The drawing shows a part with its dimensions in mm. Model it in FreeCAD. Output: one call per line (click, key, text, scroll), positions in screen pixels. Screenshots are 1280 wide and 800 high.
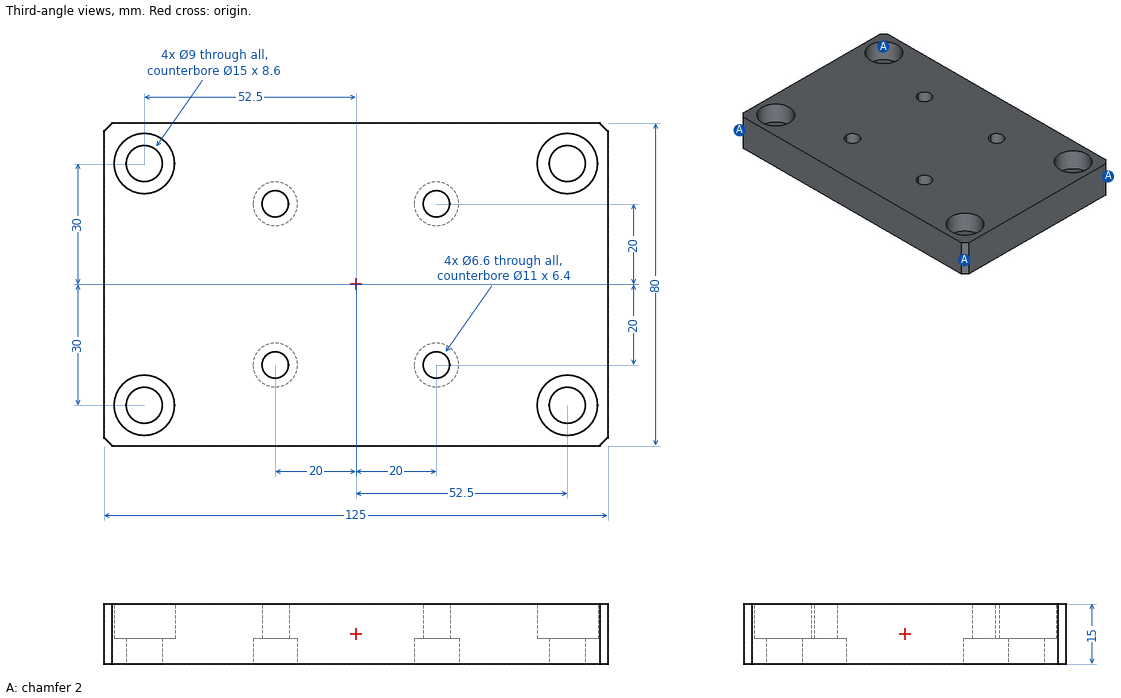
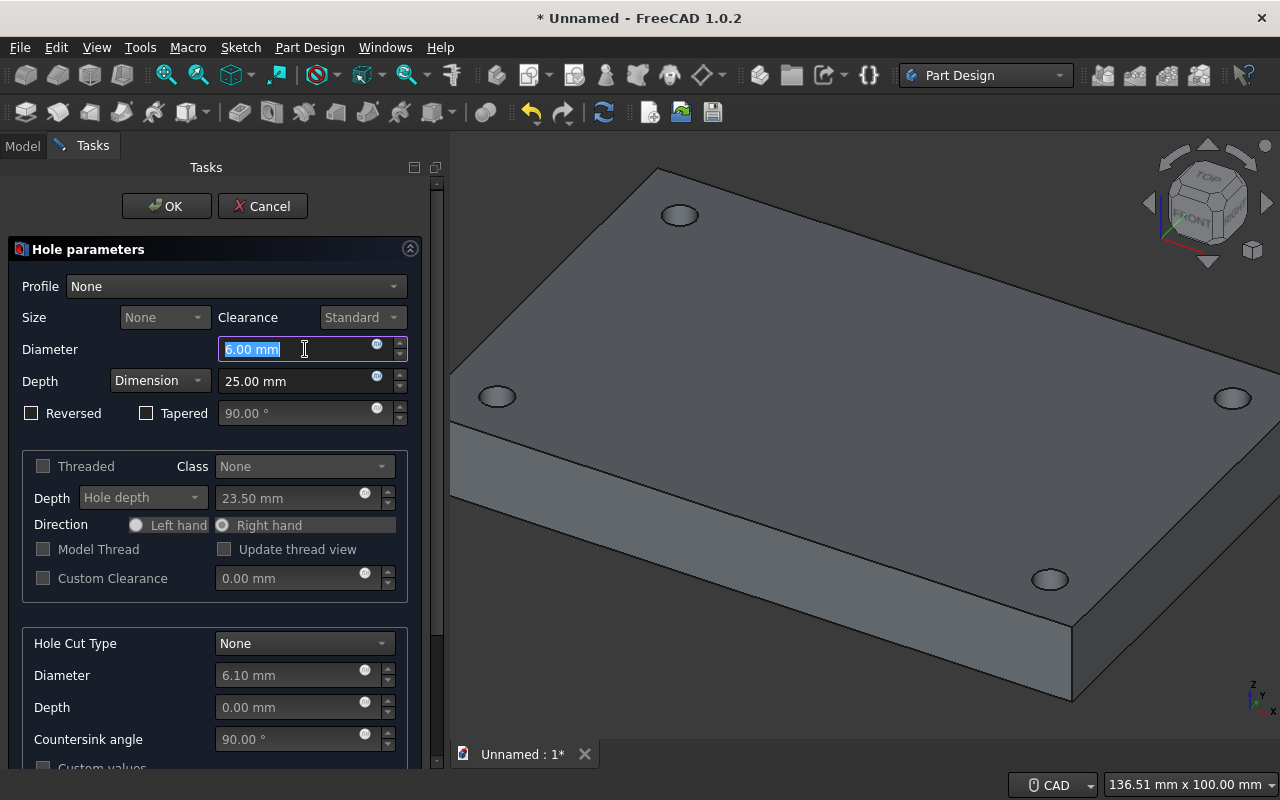
text(9)
key(Tab)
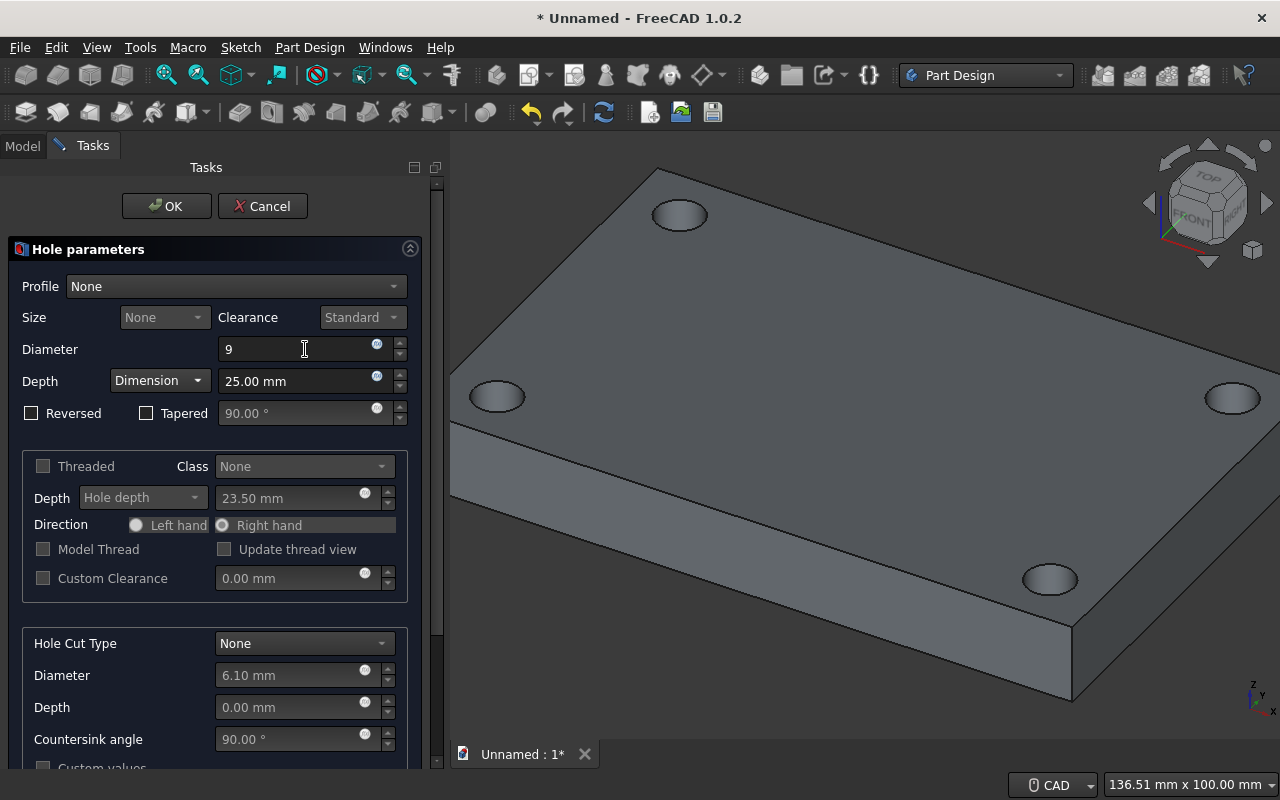
click(161, 380)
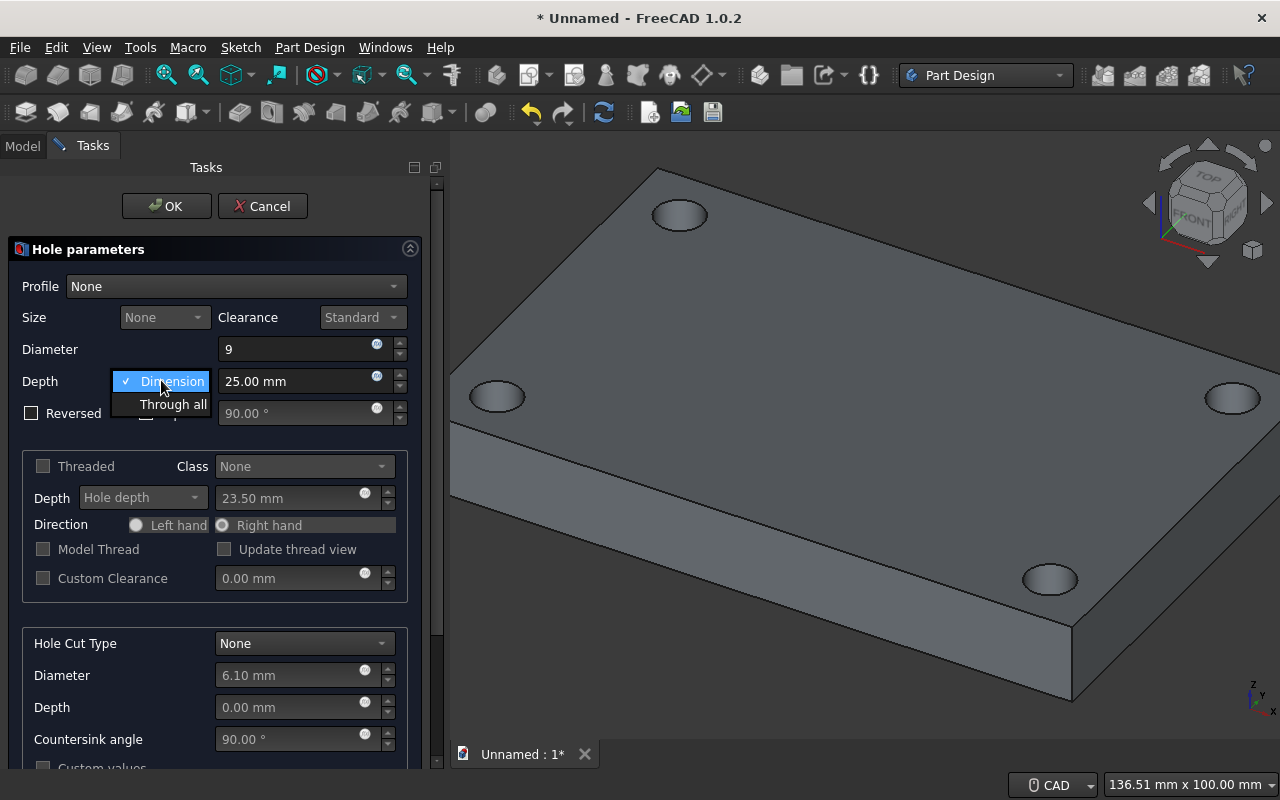
click(160, 404)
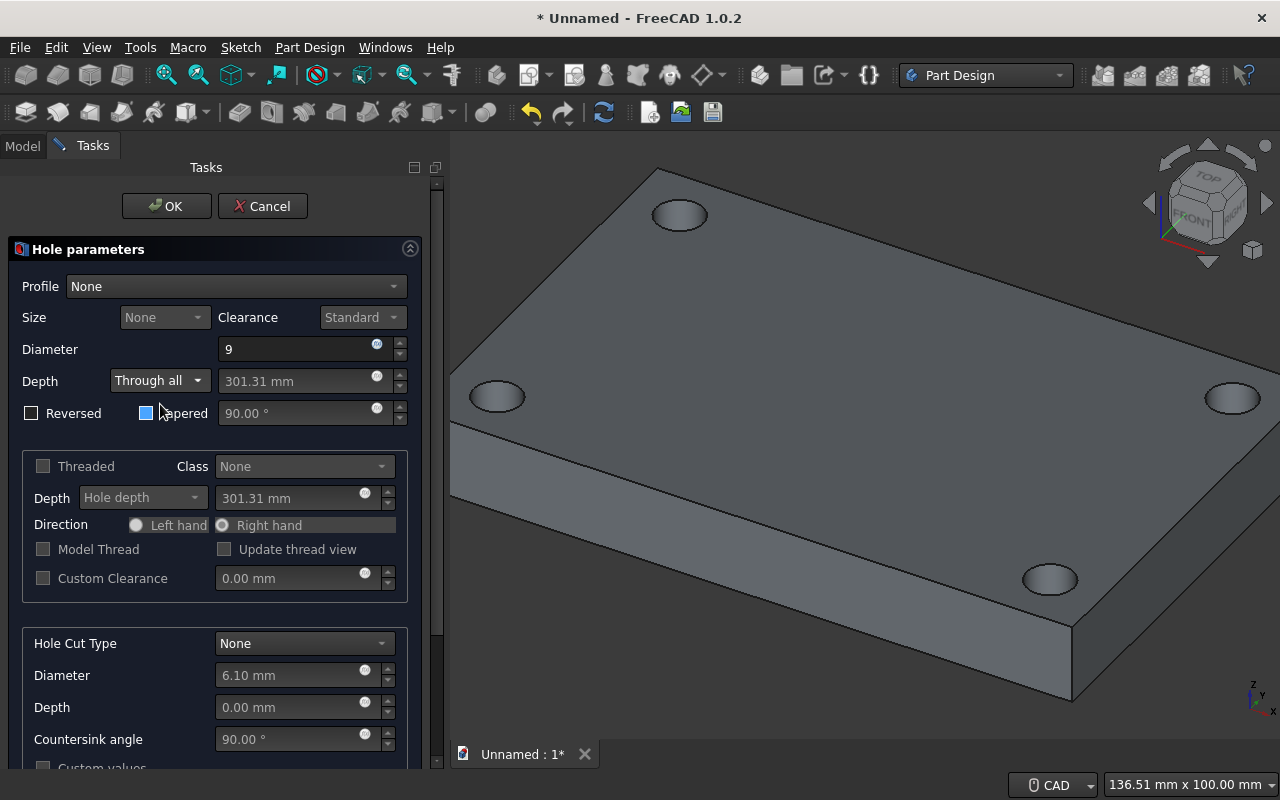
click(306, 644)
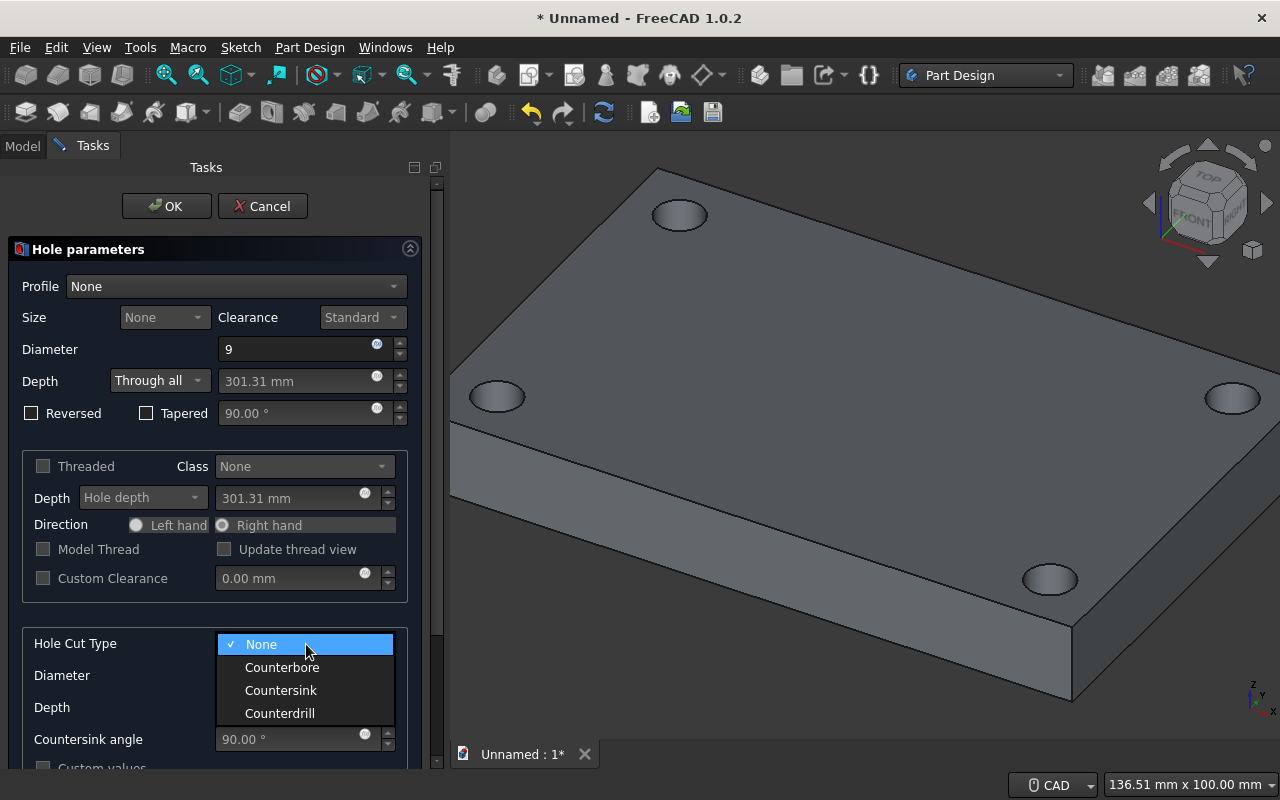
click(304, 668)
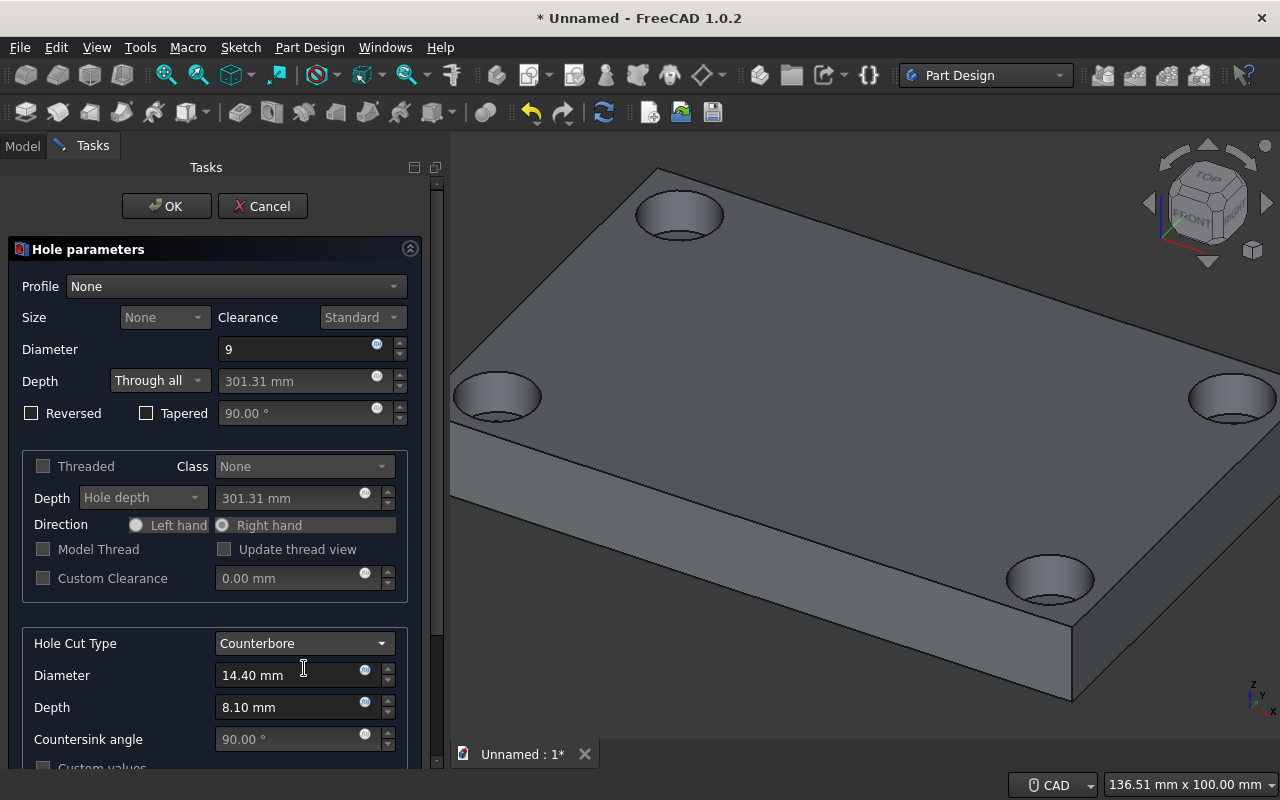
triple_click(298, 675)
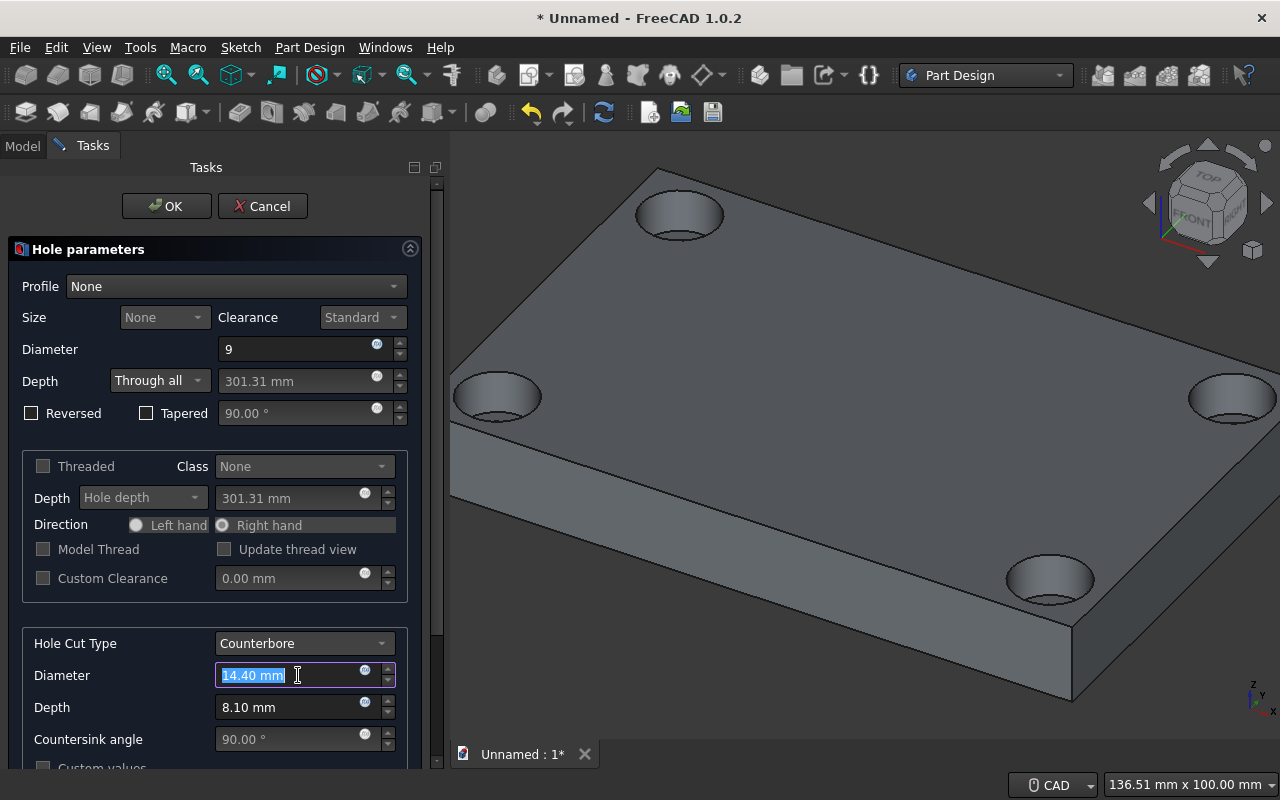
text(15)
key(Tab)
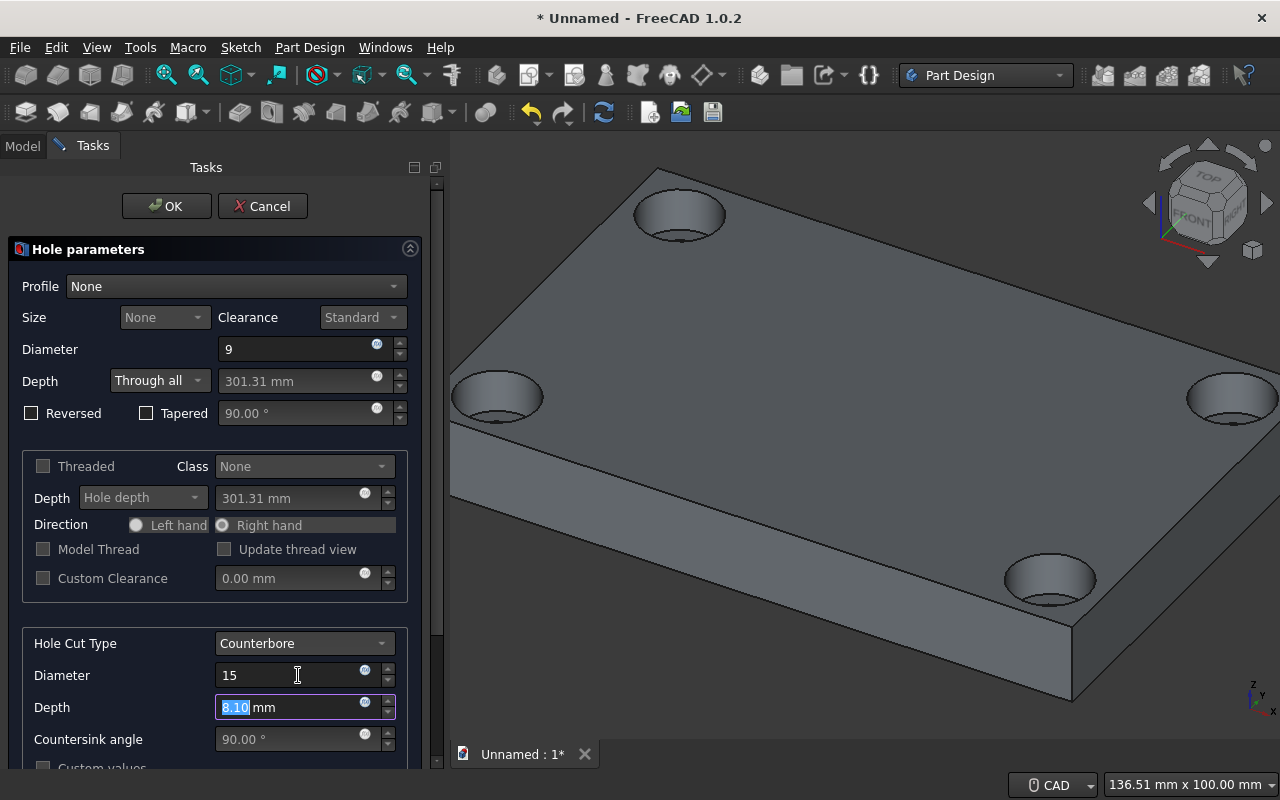
text(8.6)
key(Tab)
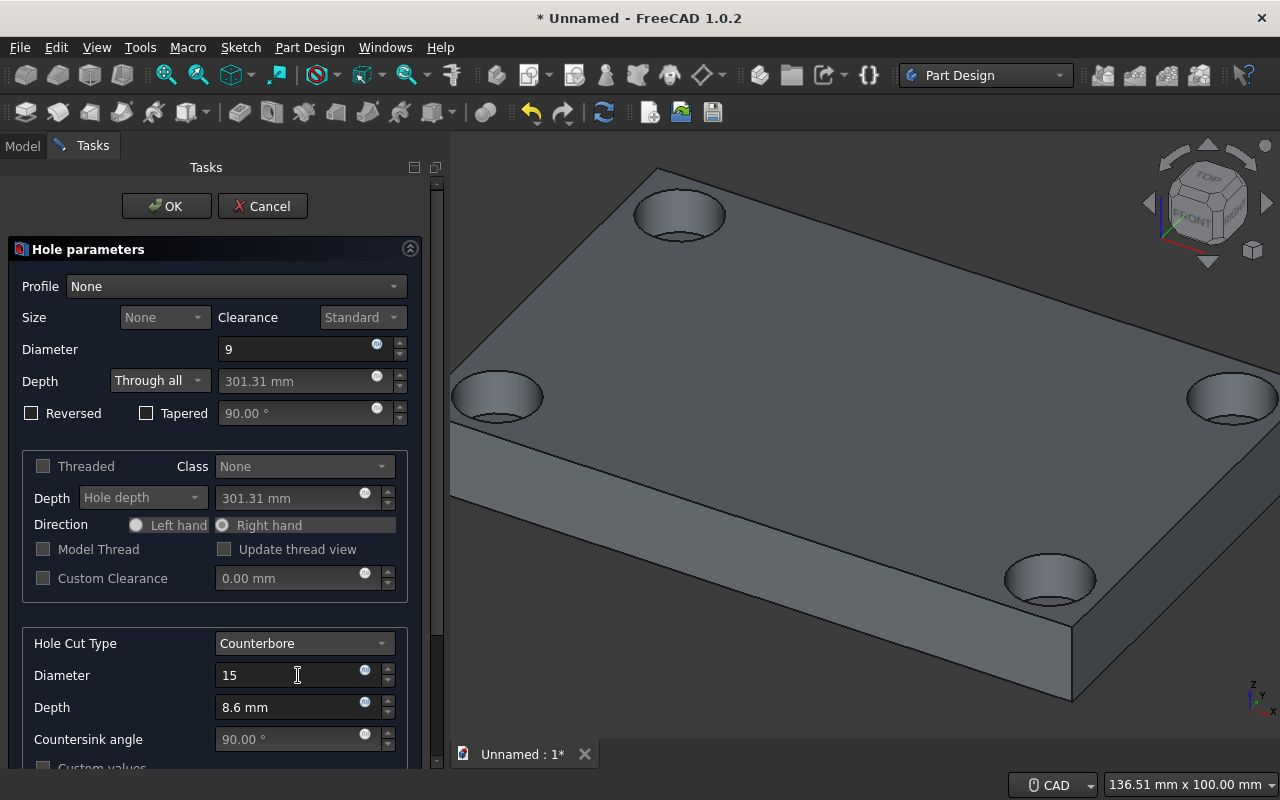
click(167, 206)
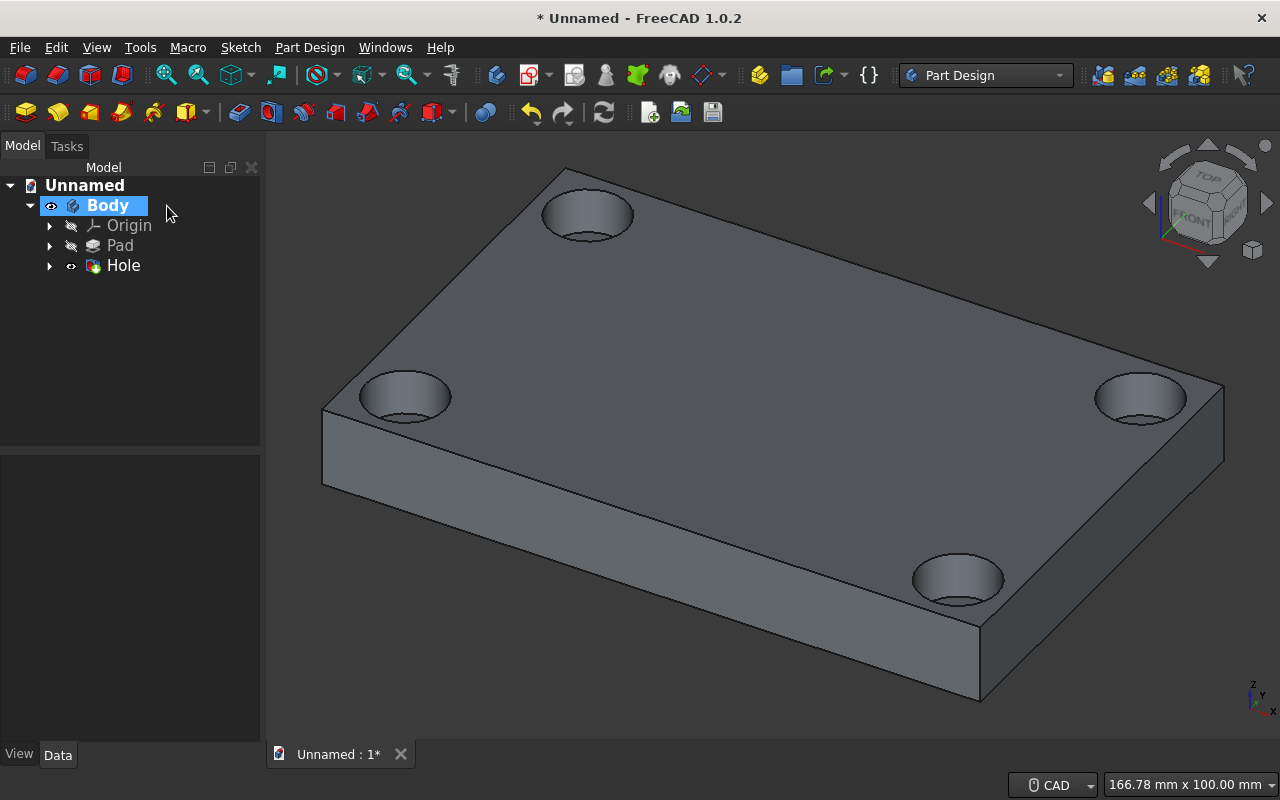
key(5)